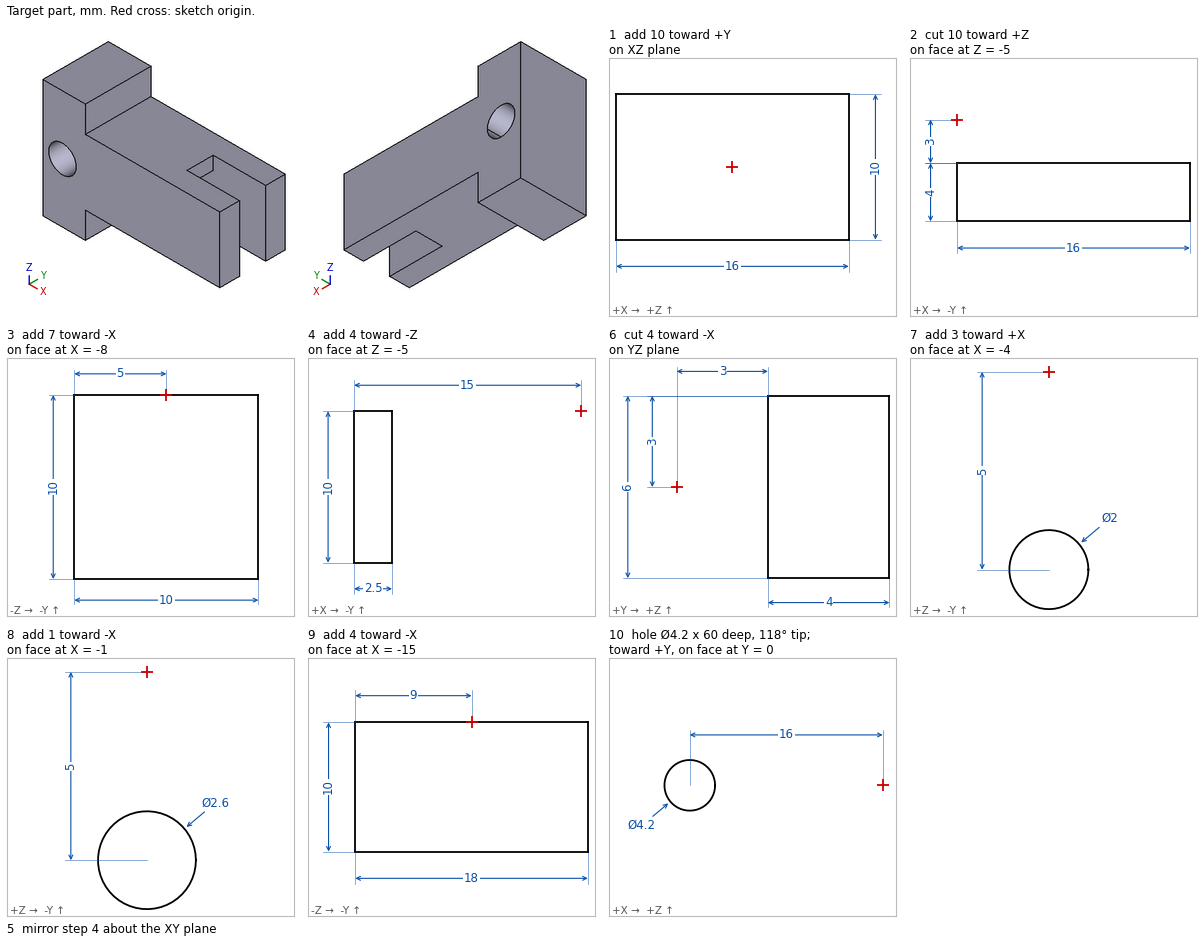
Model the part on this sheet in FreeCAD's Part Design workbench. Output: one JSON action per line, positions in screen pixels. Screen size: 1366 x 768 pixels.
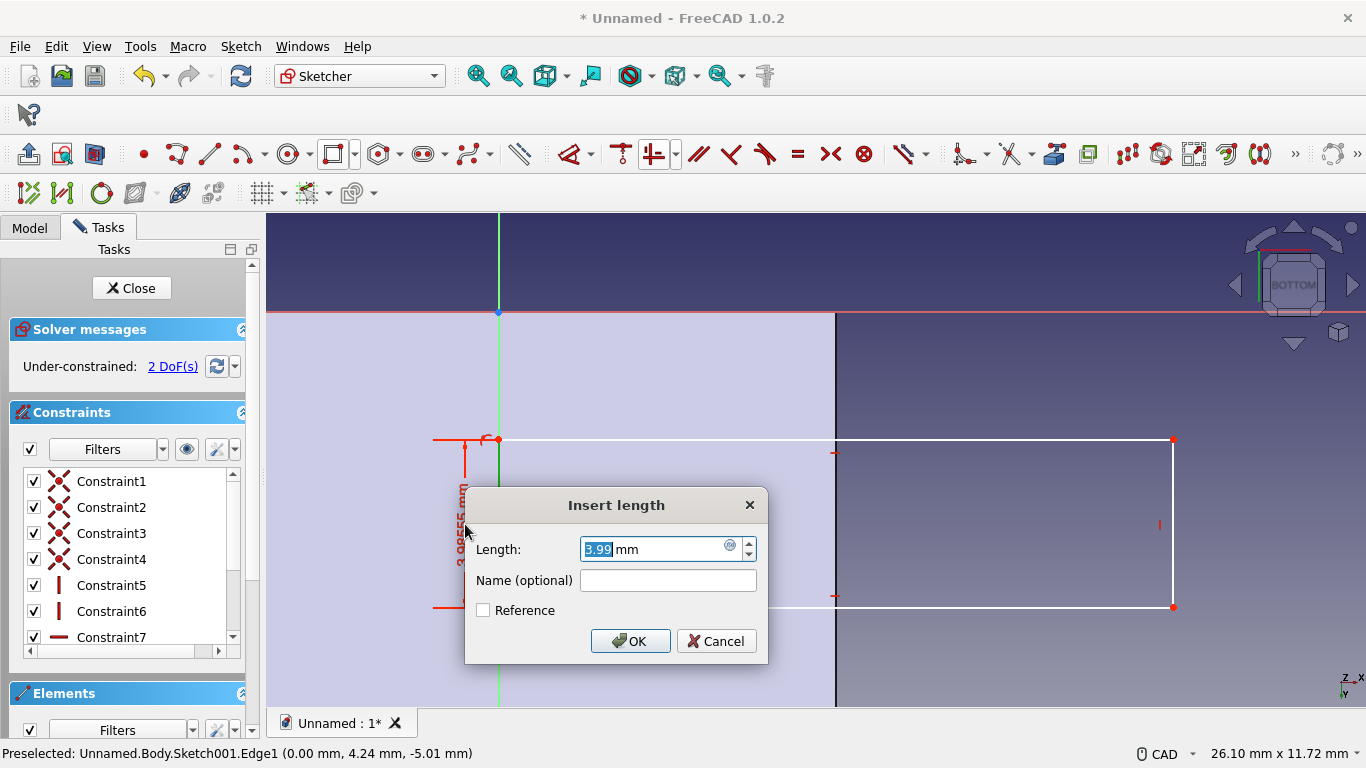
{"action": "type", "text": "4"}
{"action": "key", "text": "Return"}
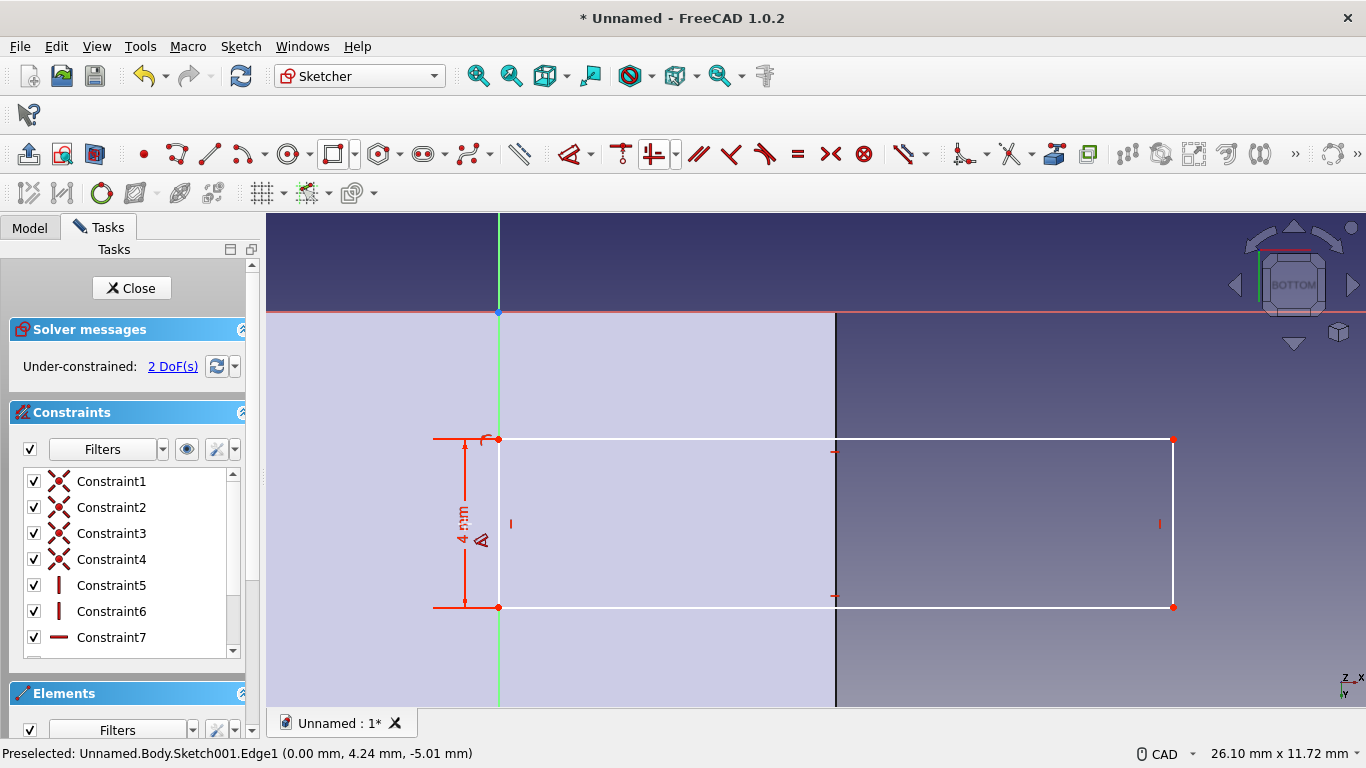
{"action": "left_click", "coordinate": [701, 608]}
{"action": "left_click", "coordinate": [836, 642]}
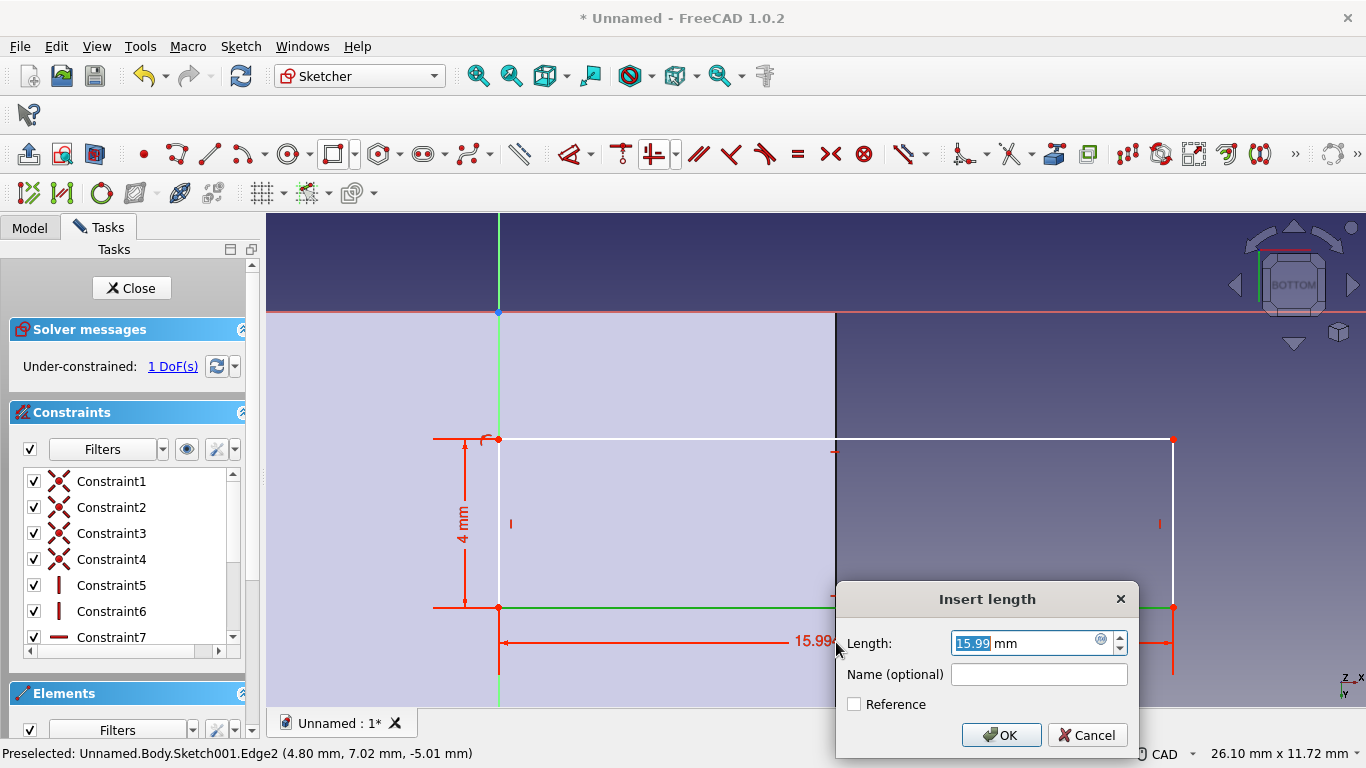
{"action": "type", "text": "16"}
{"action": "key", "text": "Return"}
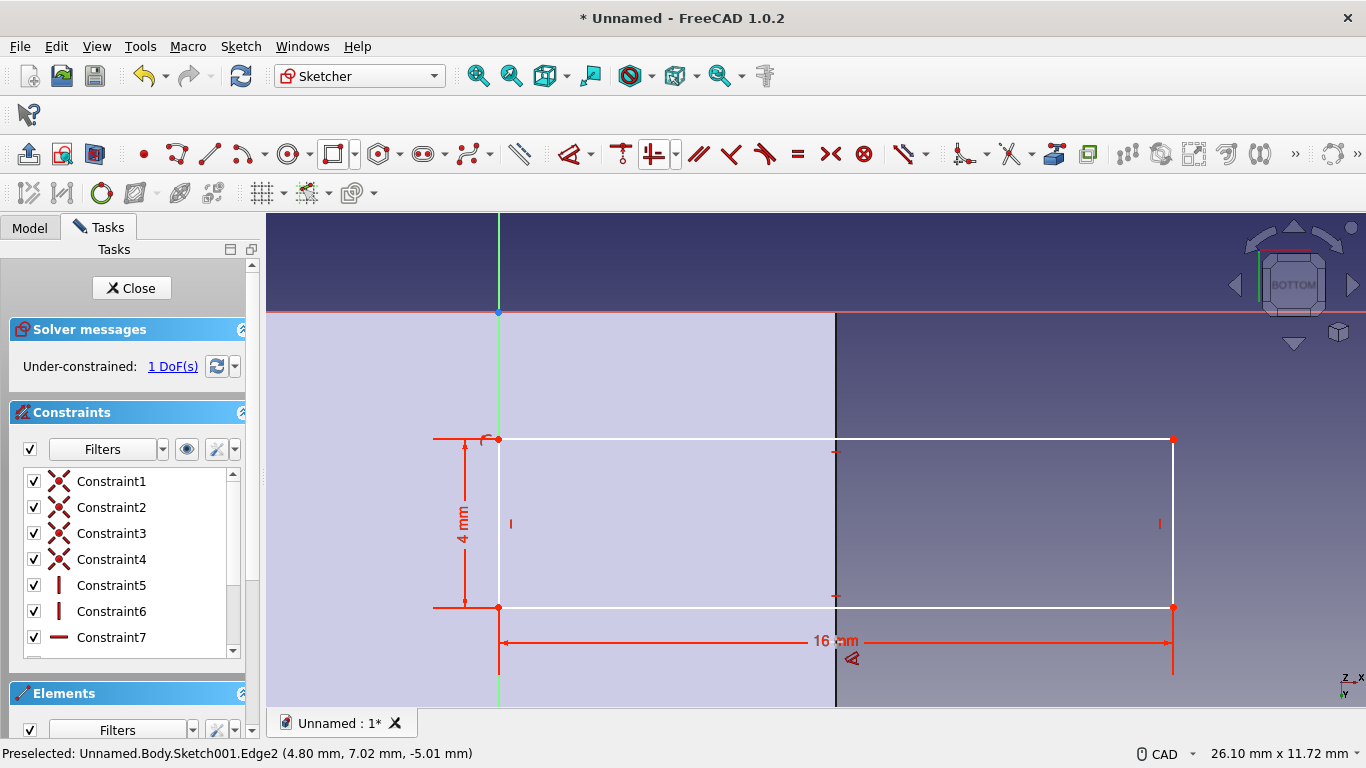
{"action": "left_click", "coordinate": [499, 439]}
{"action": "left_click", "coordinate": [465, 376]}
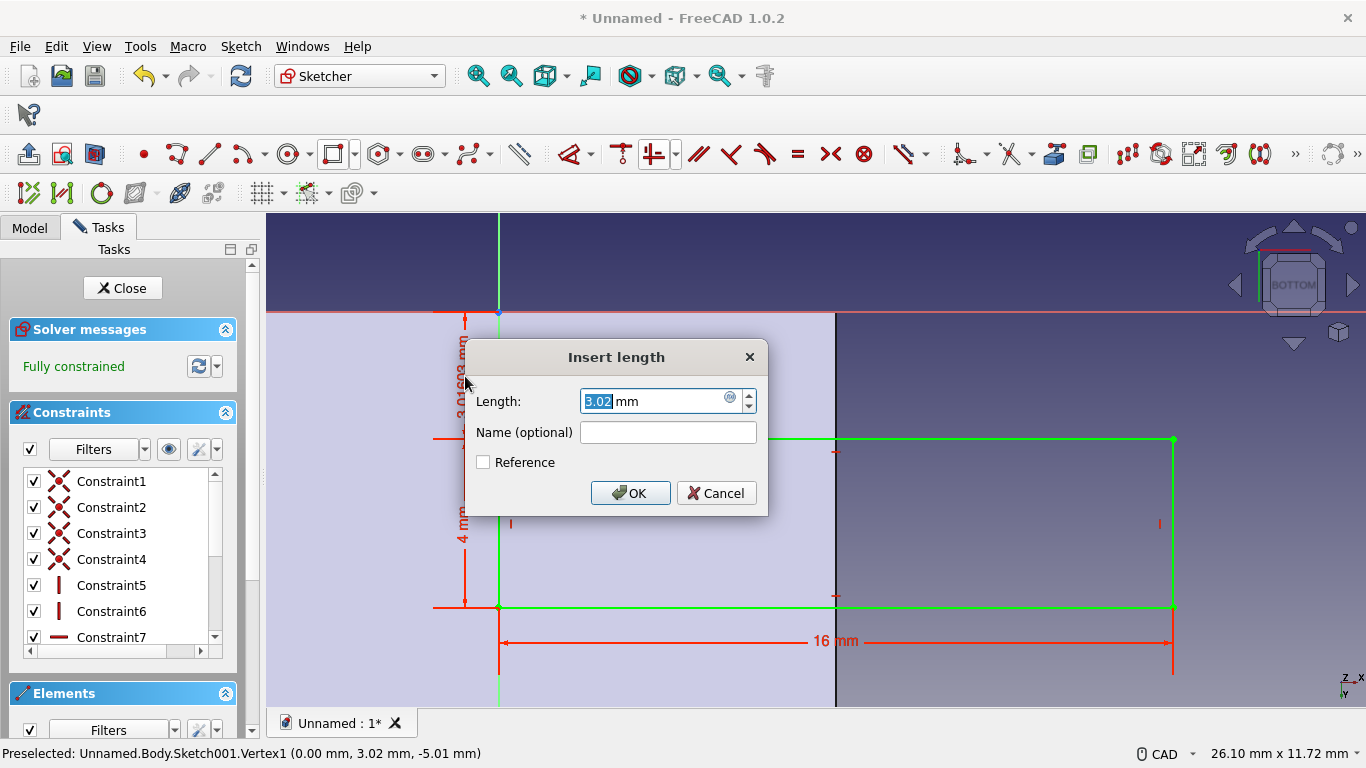
{"action": "type", "text": "3"}
{"action": "key", "text": "Return"}
{"action": "key", "text": "Escape"}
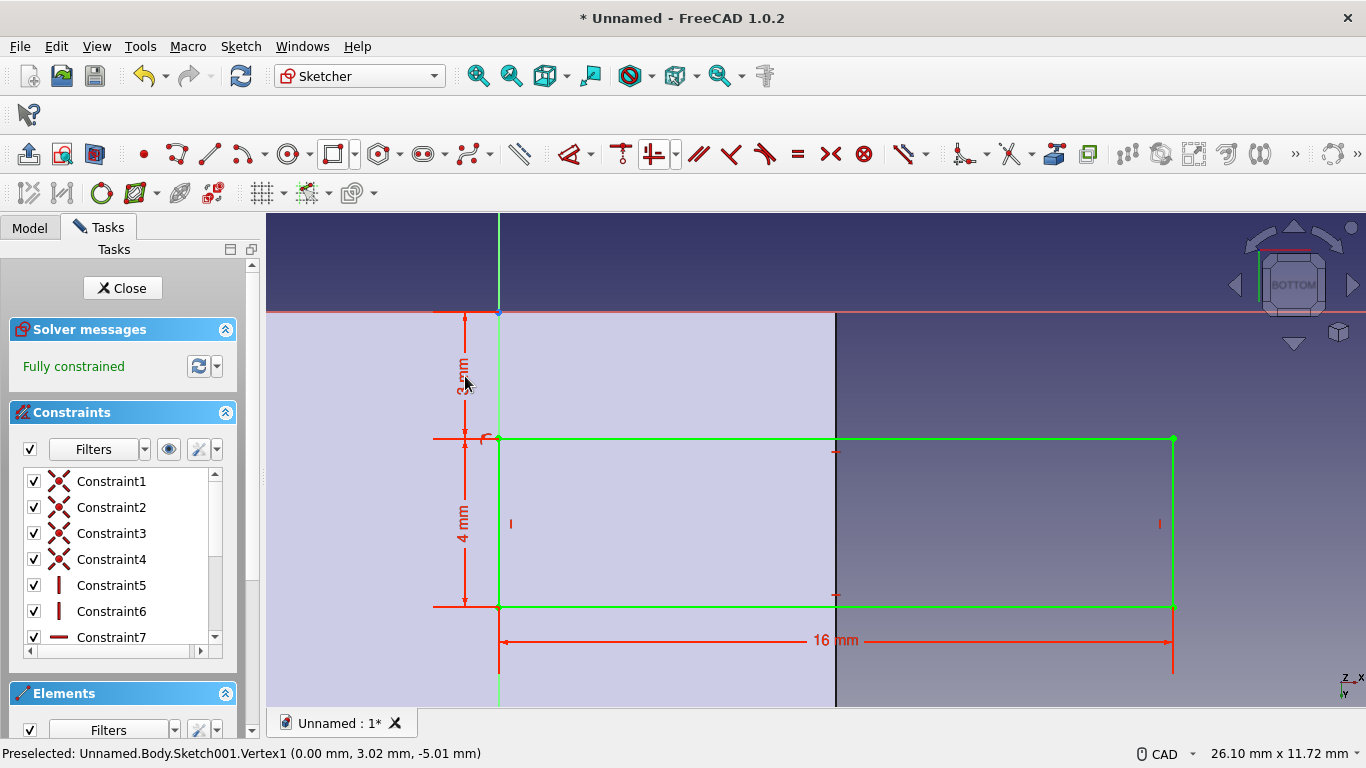
{"action": "left_click", "coordinate": [123, 288]}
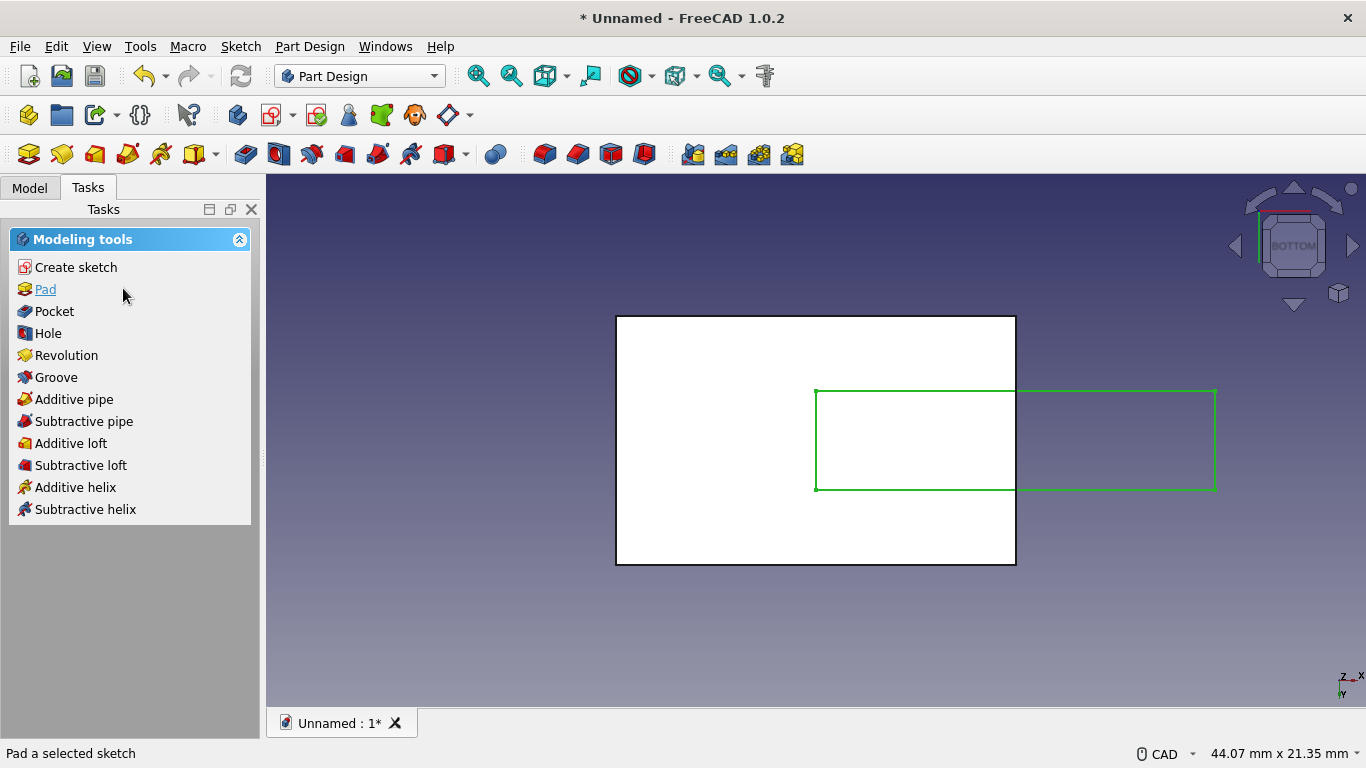
{"action": "left_click", "coordinate": [246, 154]}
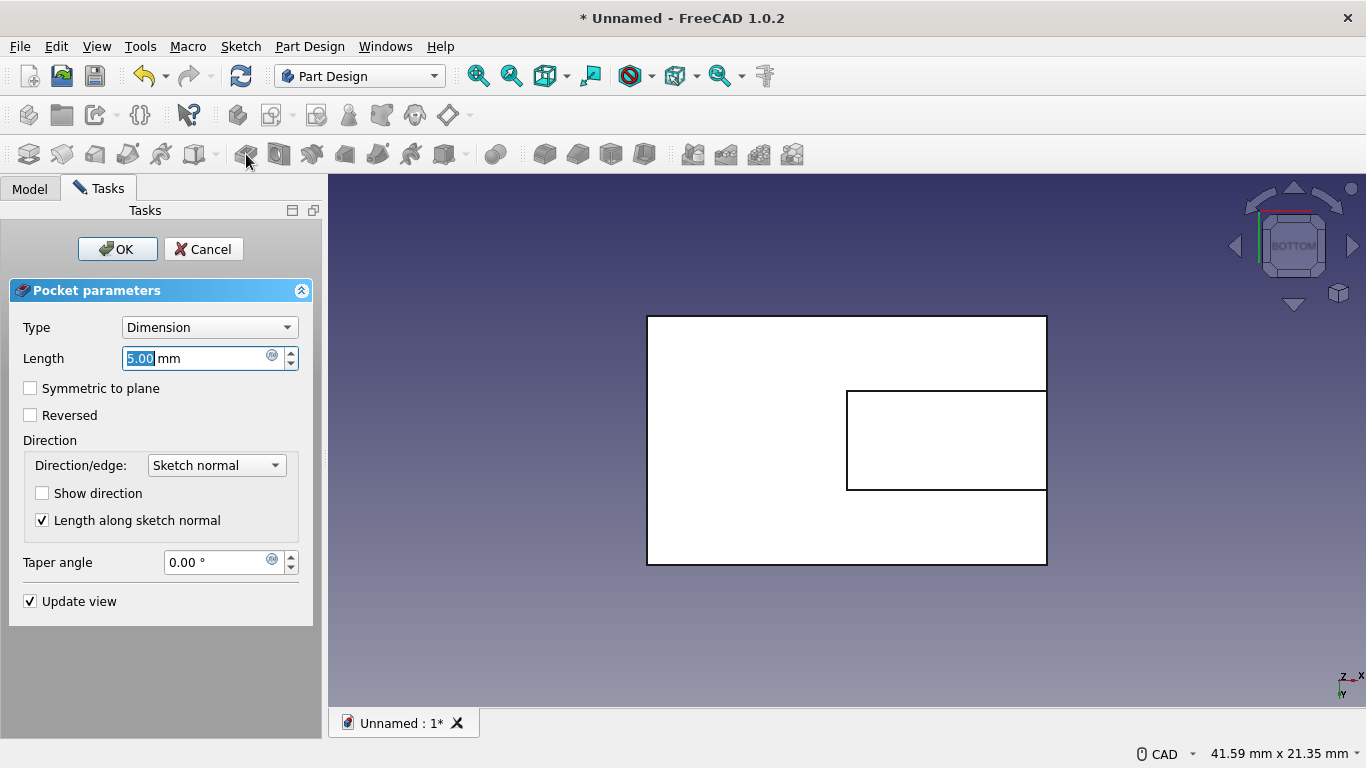
{"action": "type", "text": "10"}
{"action": "key", "text": "Tab"}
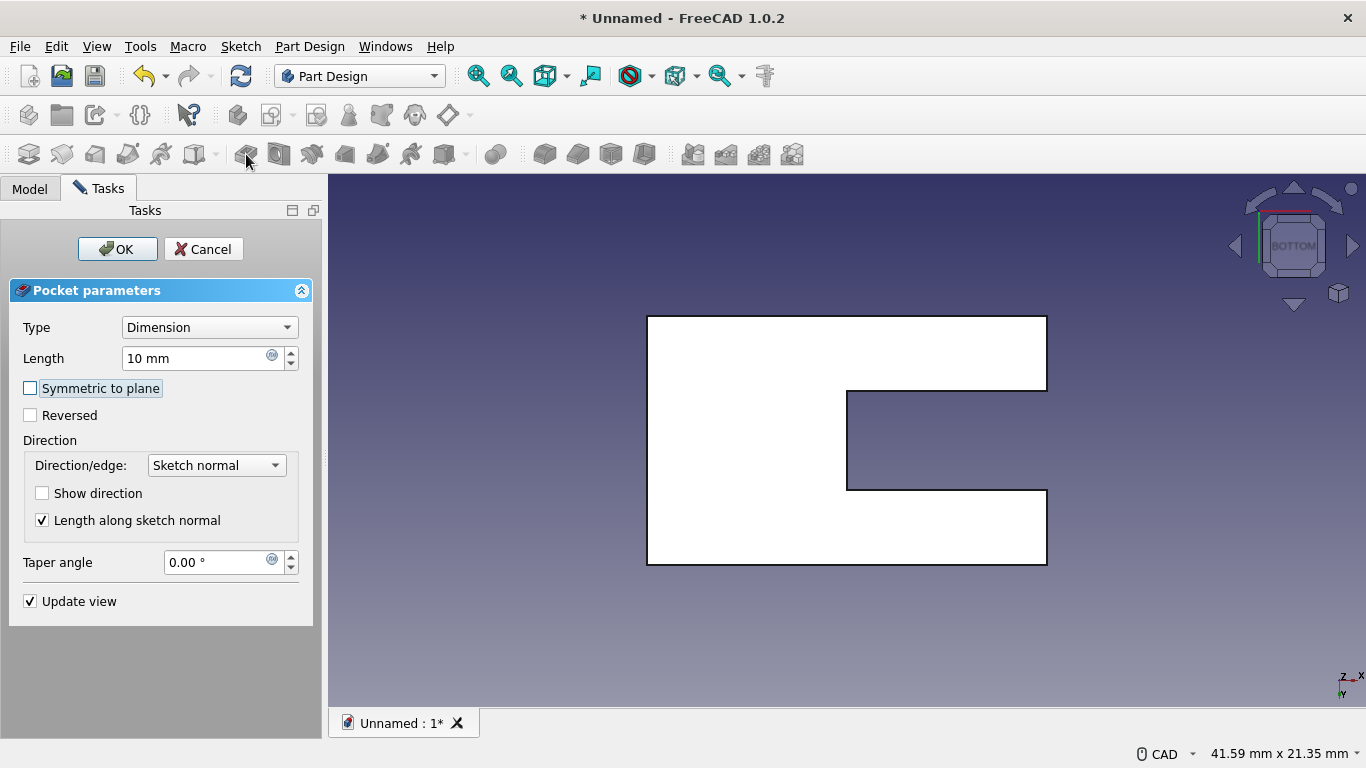
{"action": "left_click", "coordinate": [118, 249]}